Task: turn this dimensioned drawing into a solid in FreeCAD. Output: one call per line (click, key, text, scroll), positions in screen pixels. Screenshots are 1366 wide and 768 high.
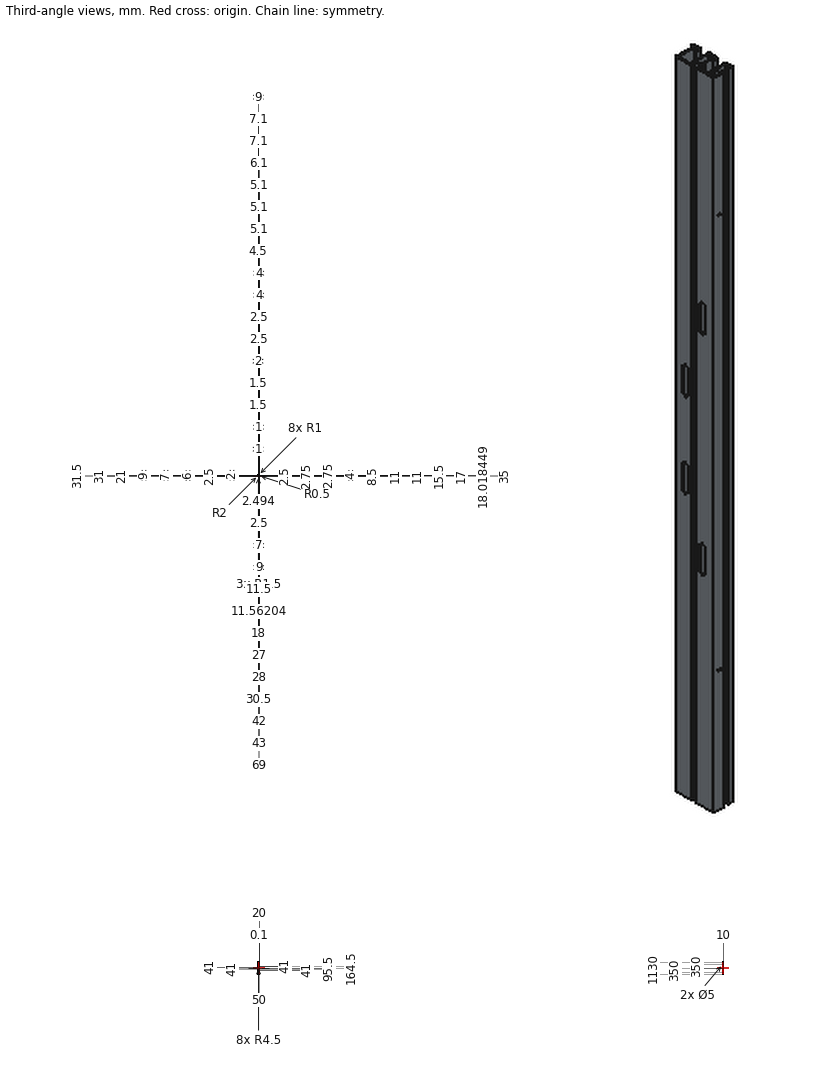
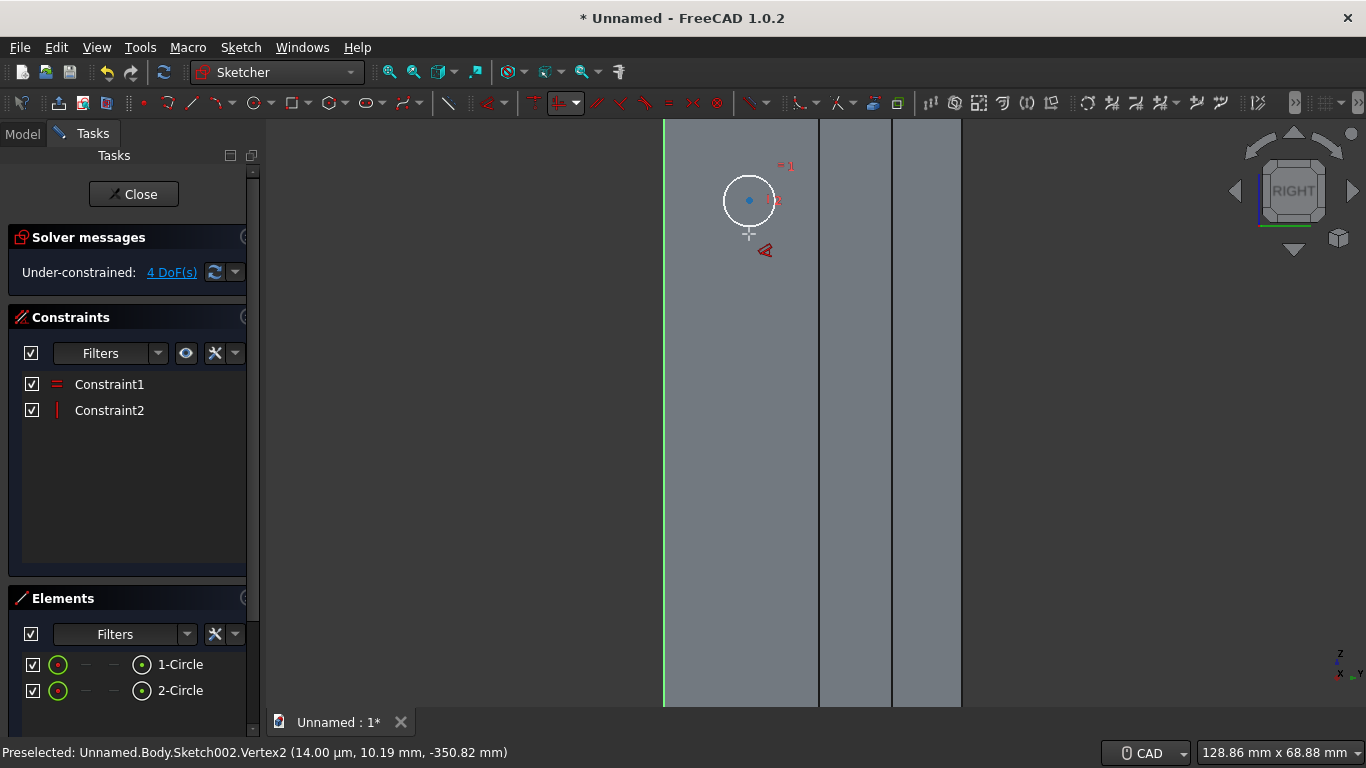
click(749, 226)
click(749, 258)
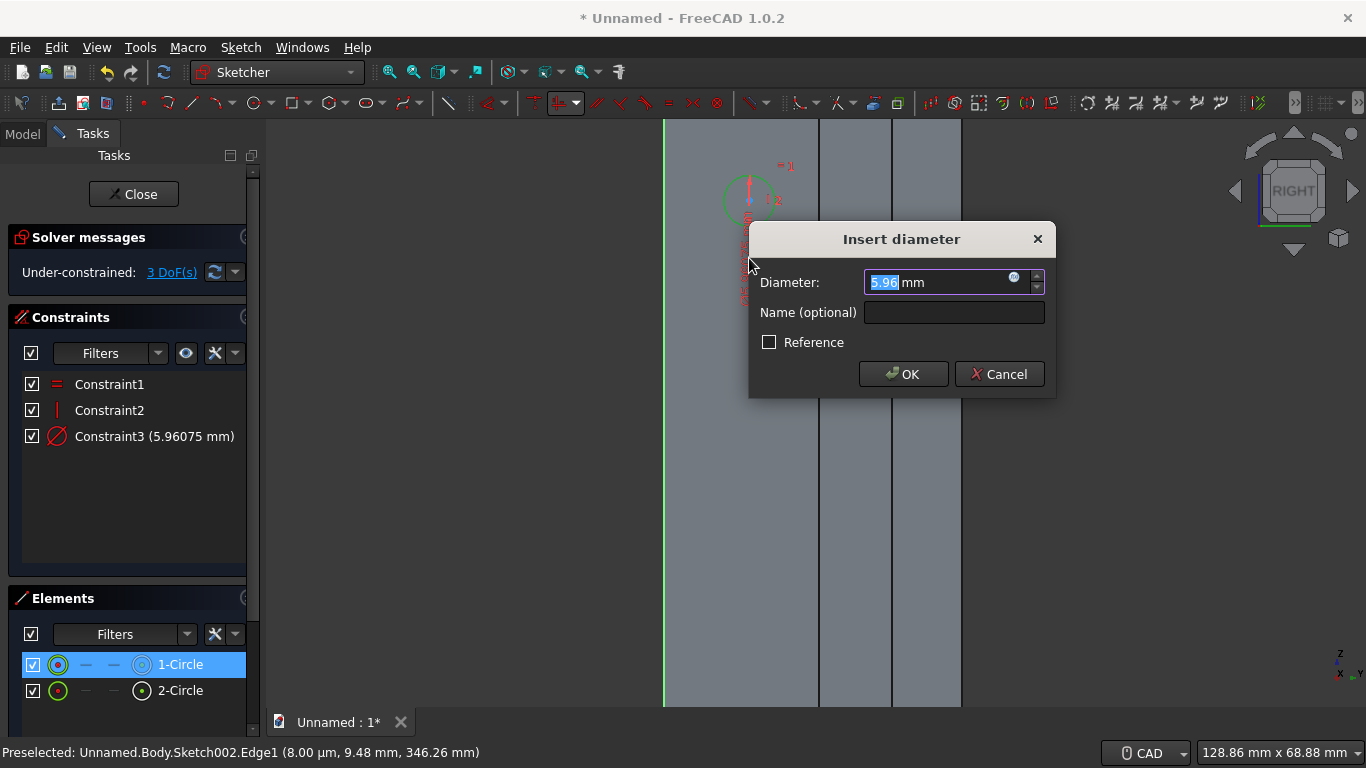
text(5)
key(Return)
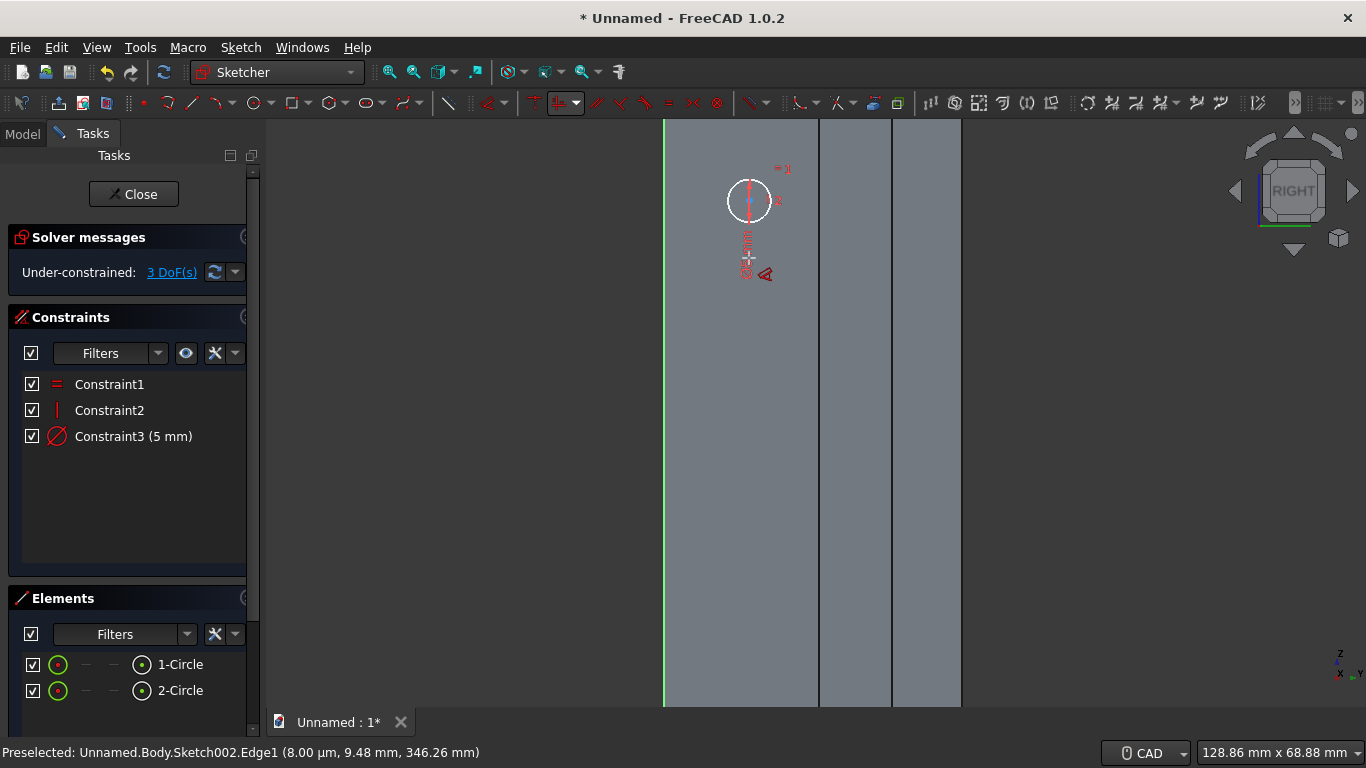
click(749, 201)
click(707, 167)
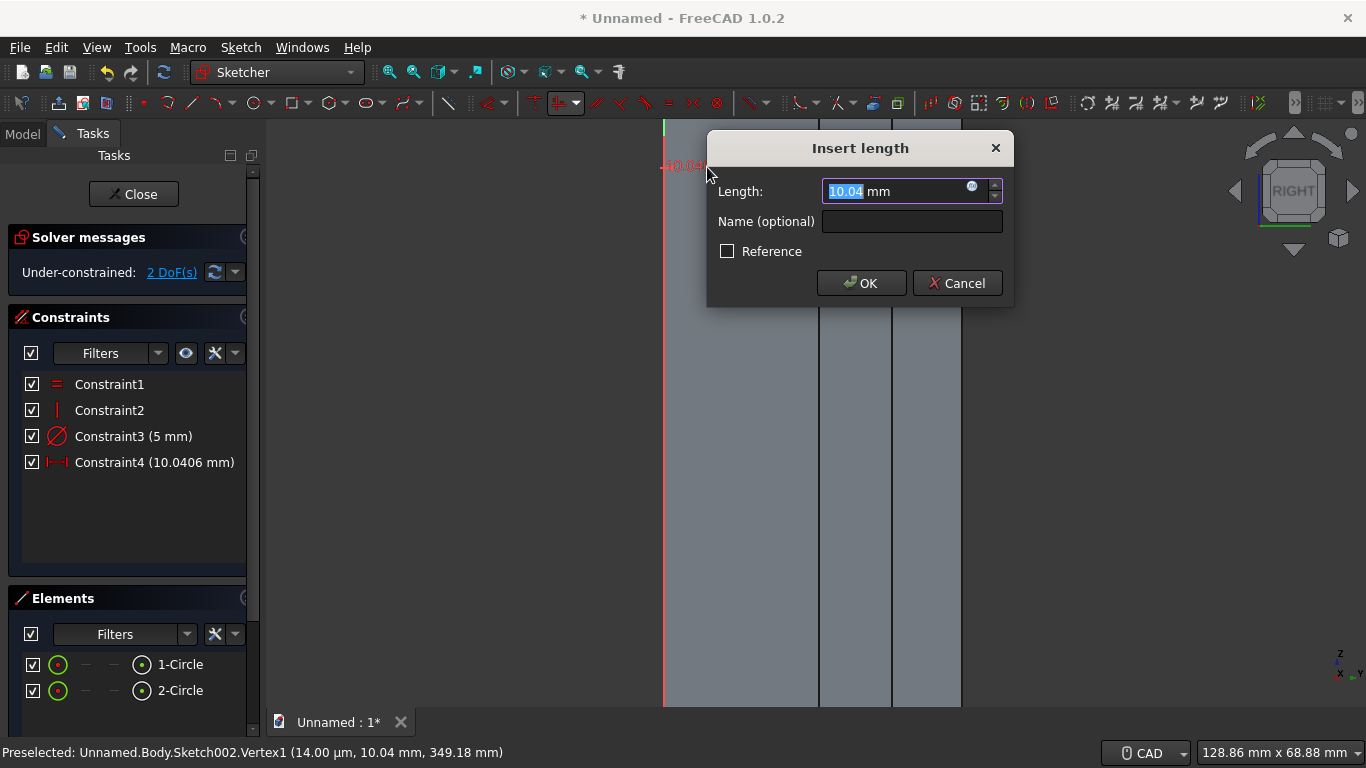
text(10)
key(Return)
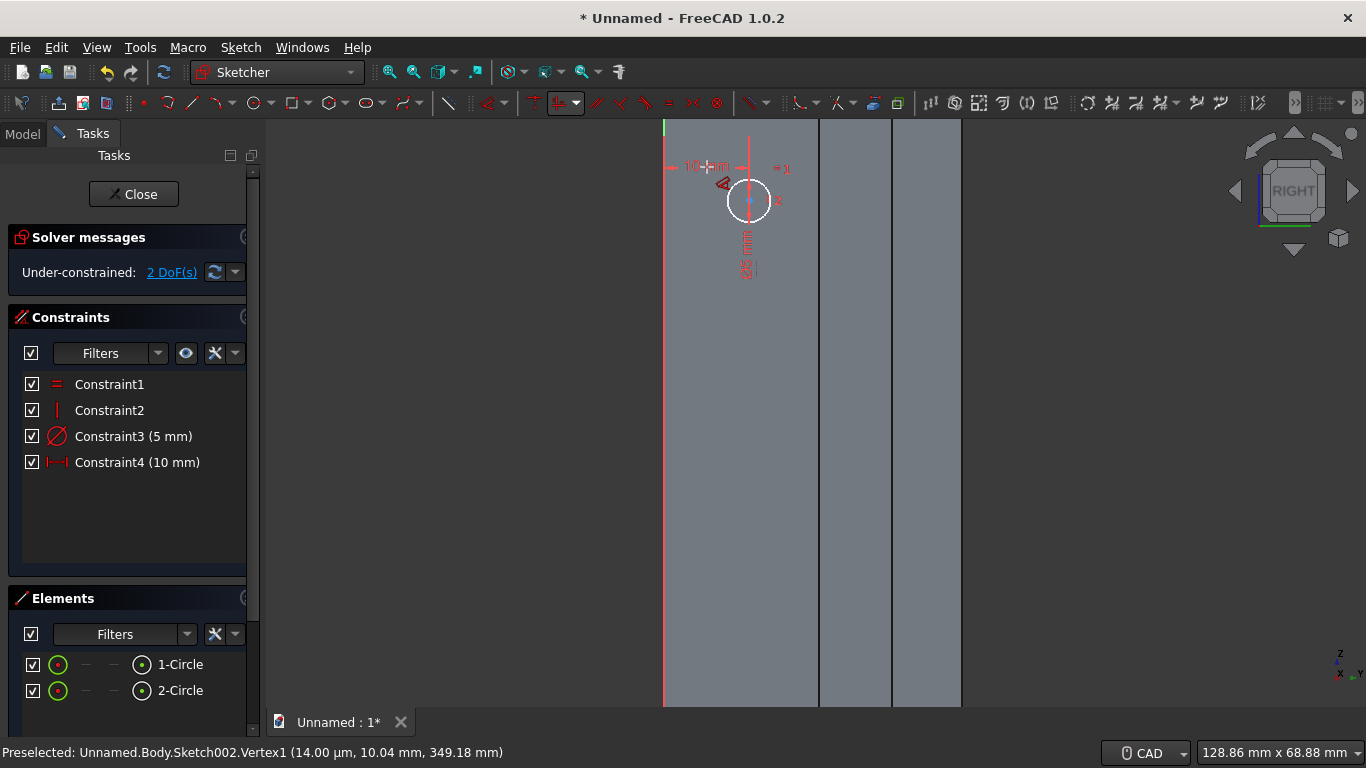
scroll(749, 234, down, 14)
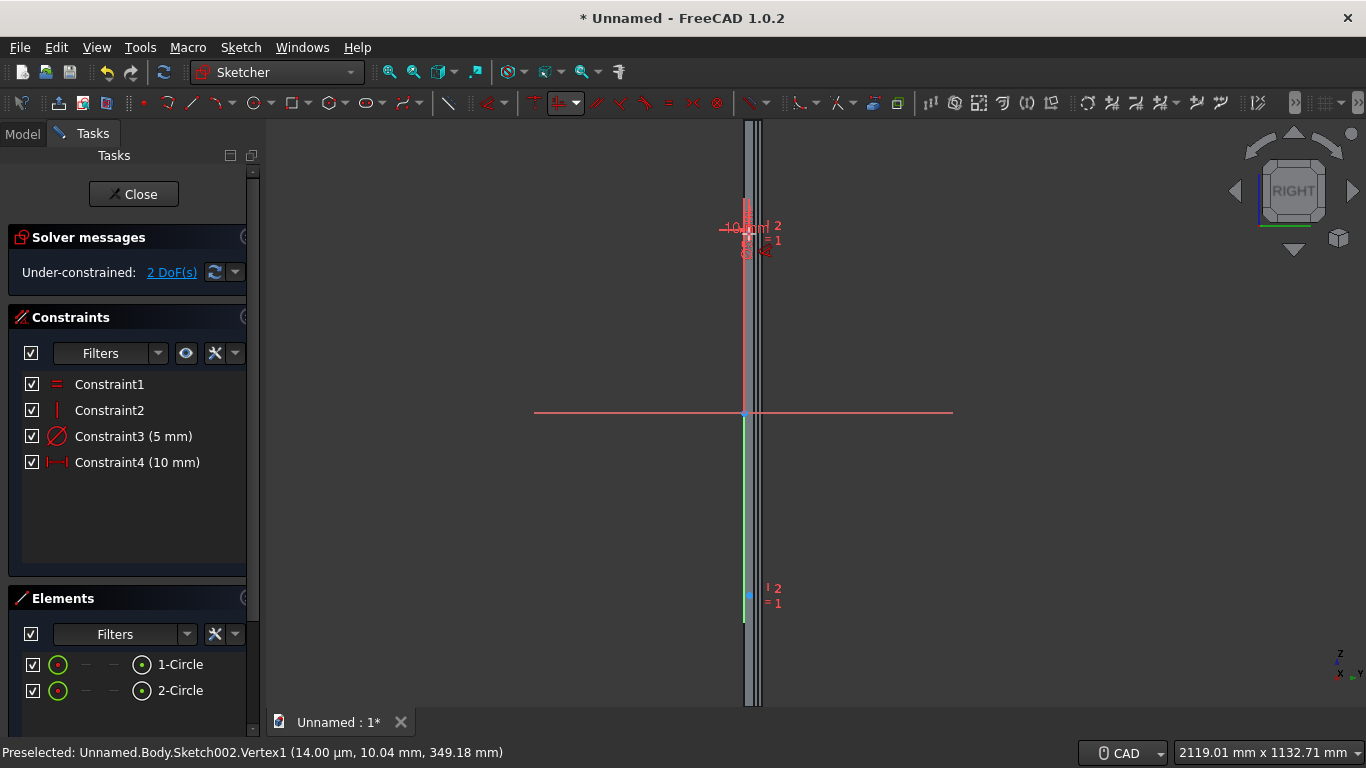
click(749, 232)
click(710, 323)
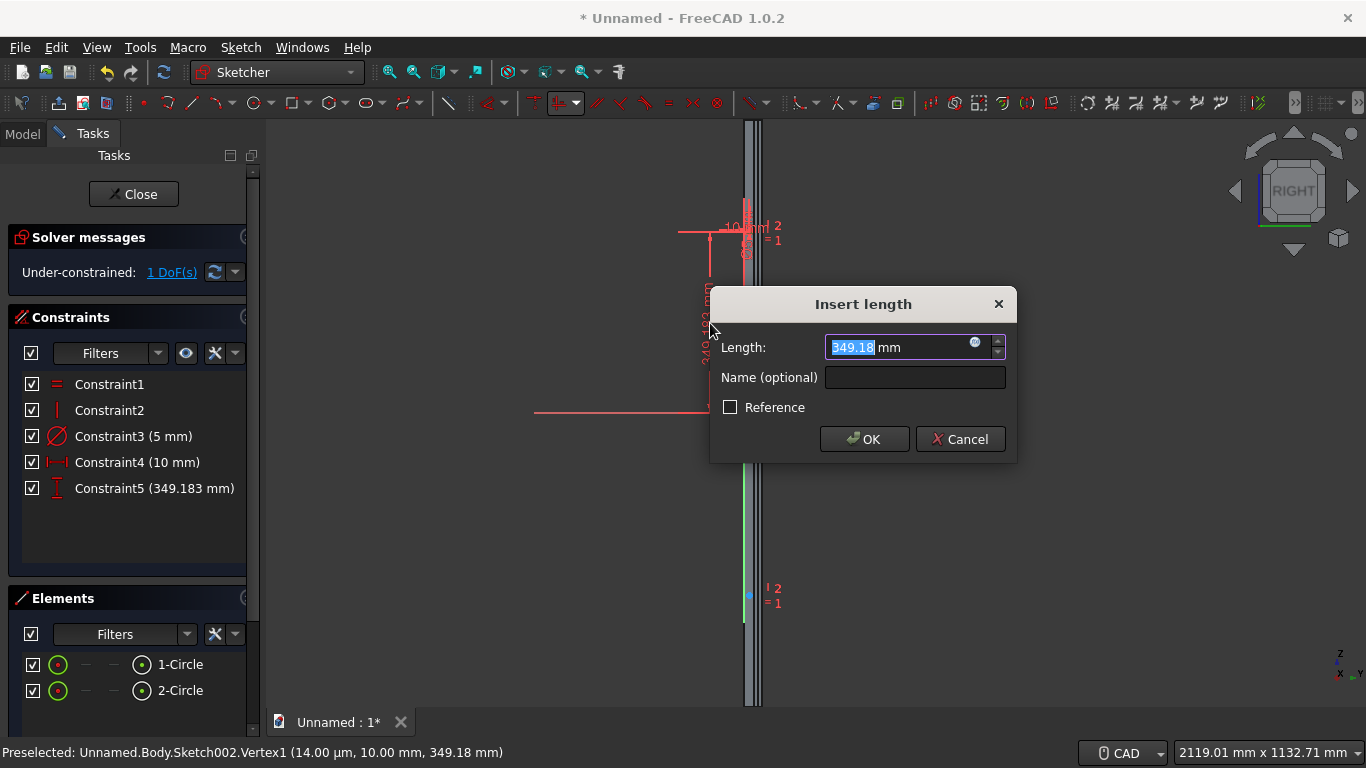
text(350)
key(Return)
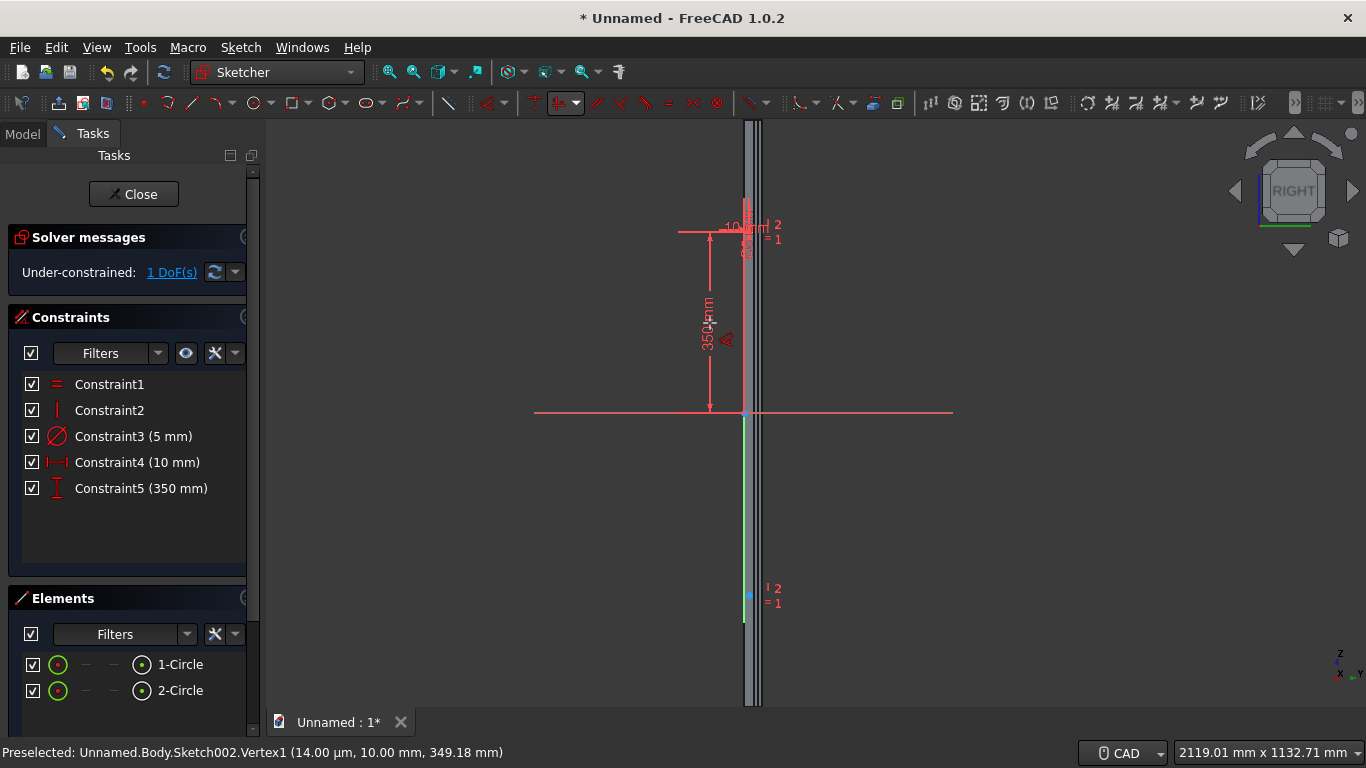
click(749, 596)
click(710, 504)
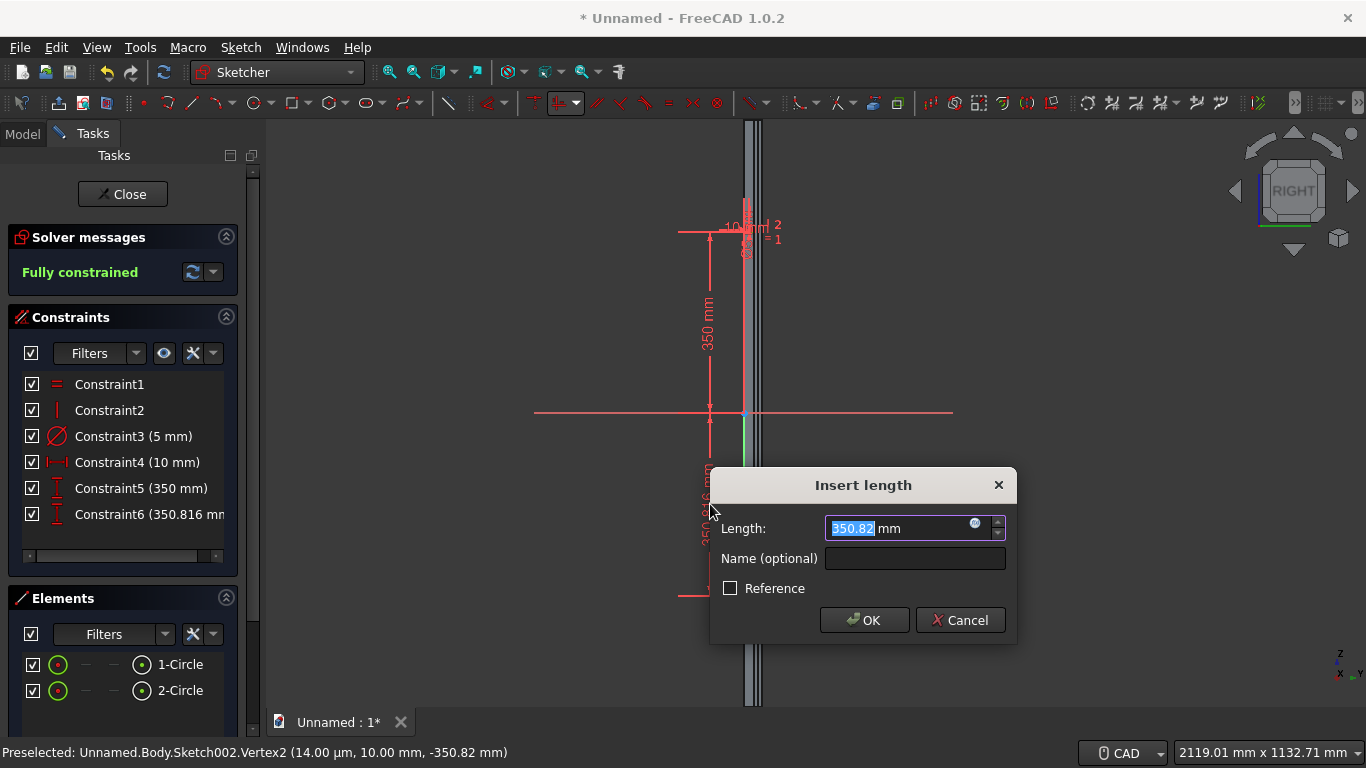
text(350)
key(Return)
key(Escape)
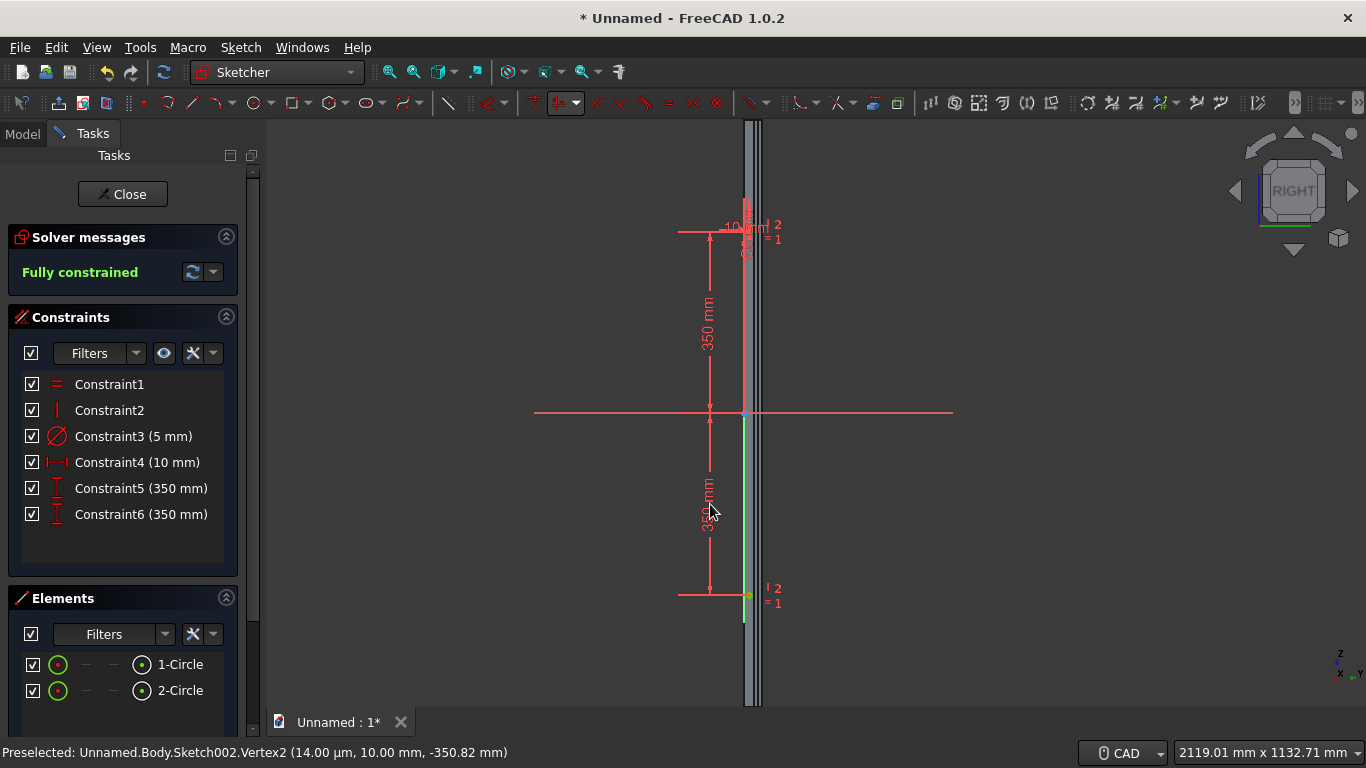
click(123, 194)